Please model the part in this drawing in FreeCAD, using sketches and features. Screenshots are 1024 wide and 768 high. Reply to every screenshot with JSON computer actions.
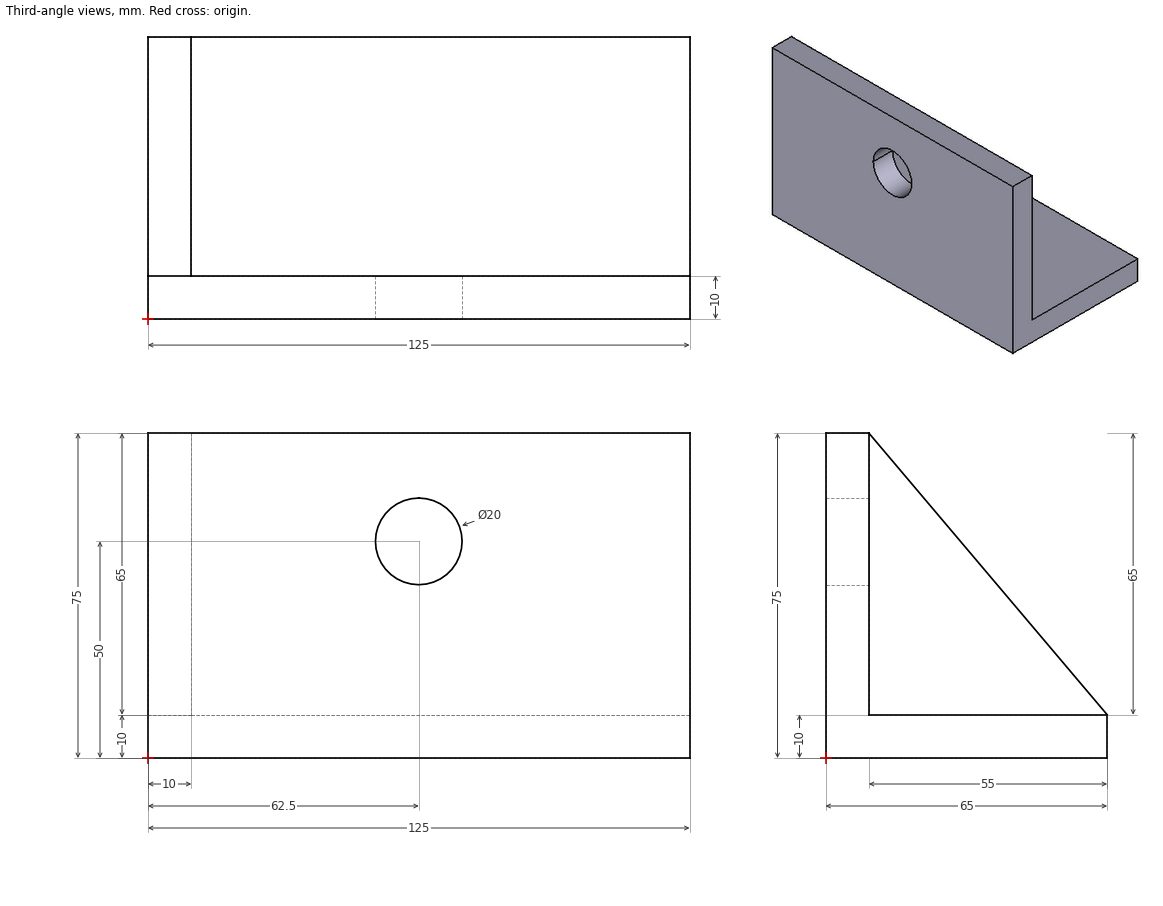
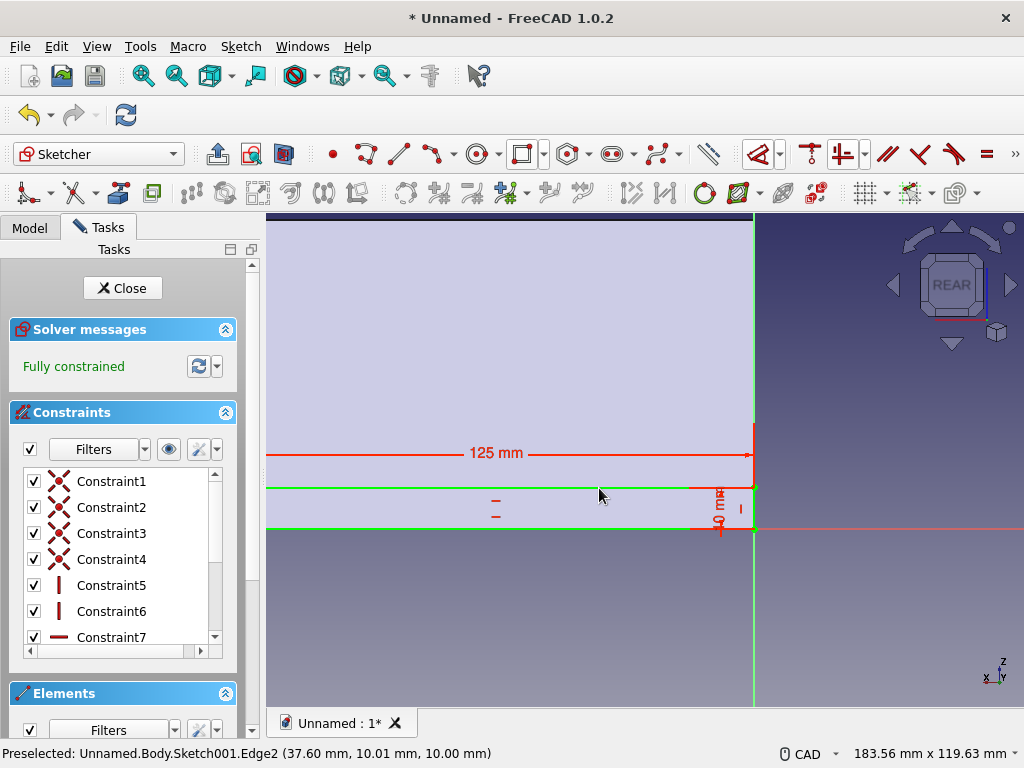
{"action": "left_click", "coordinate": [123, 288]}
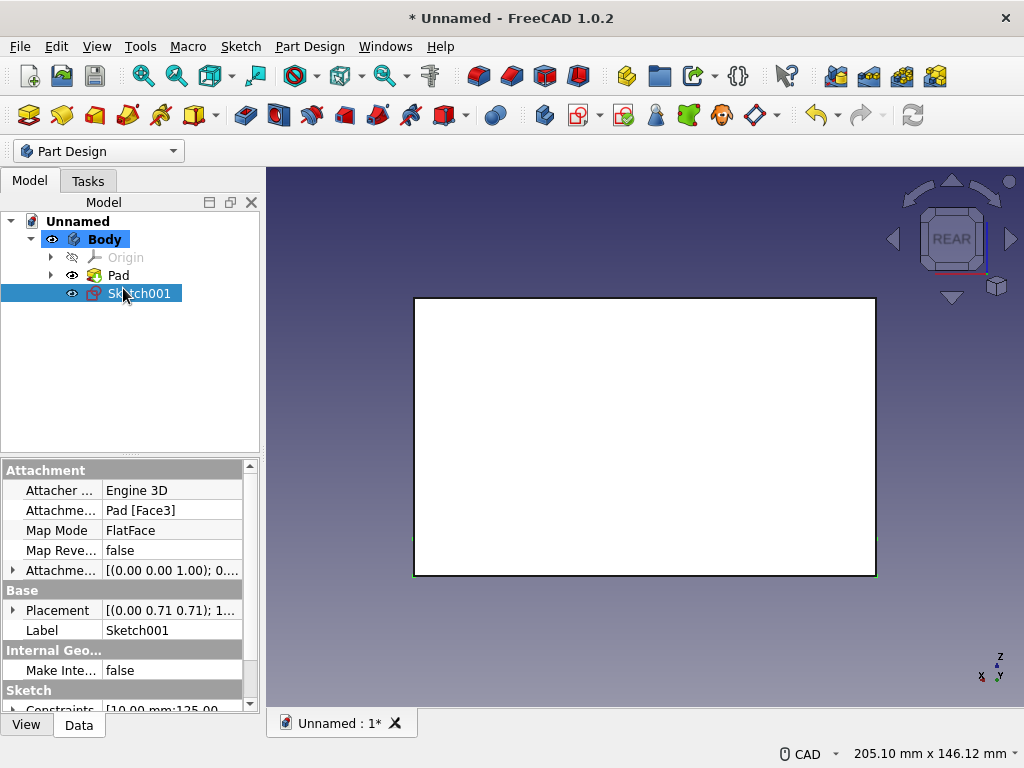
{"action": "left_click", "coordinate": [29, 116]}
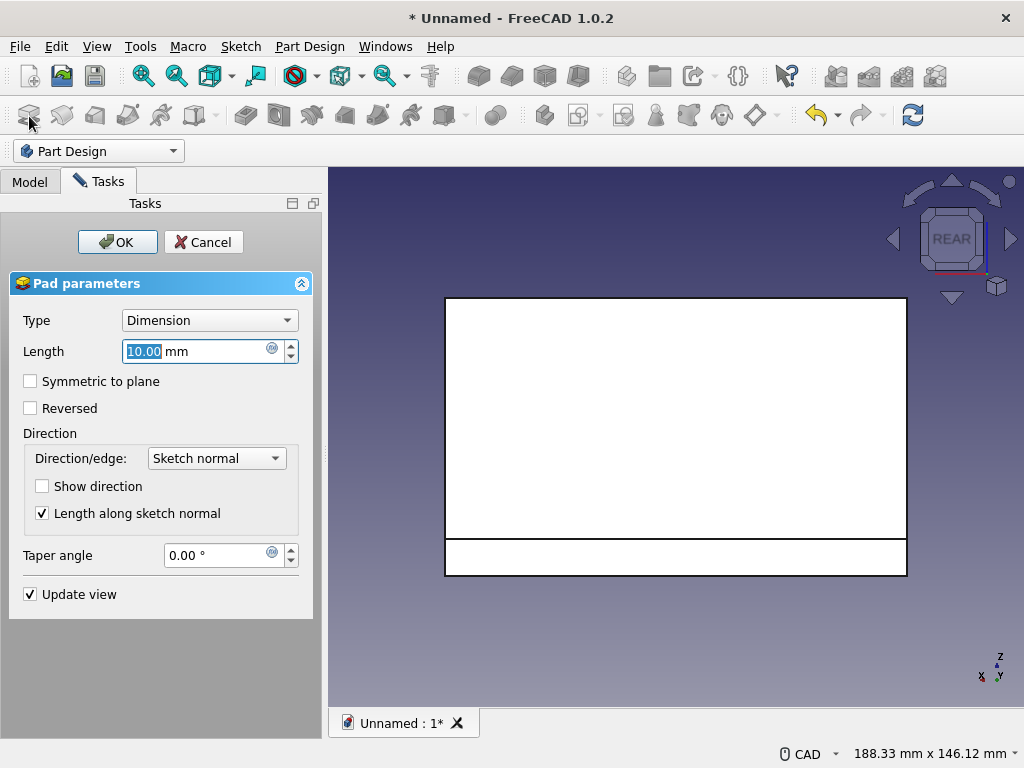
{"action": "type", "text": "55"}
{"action": "key", "text": "Tab"}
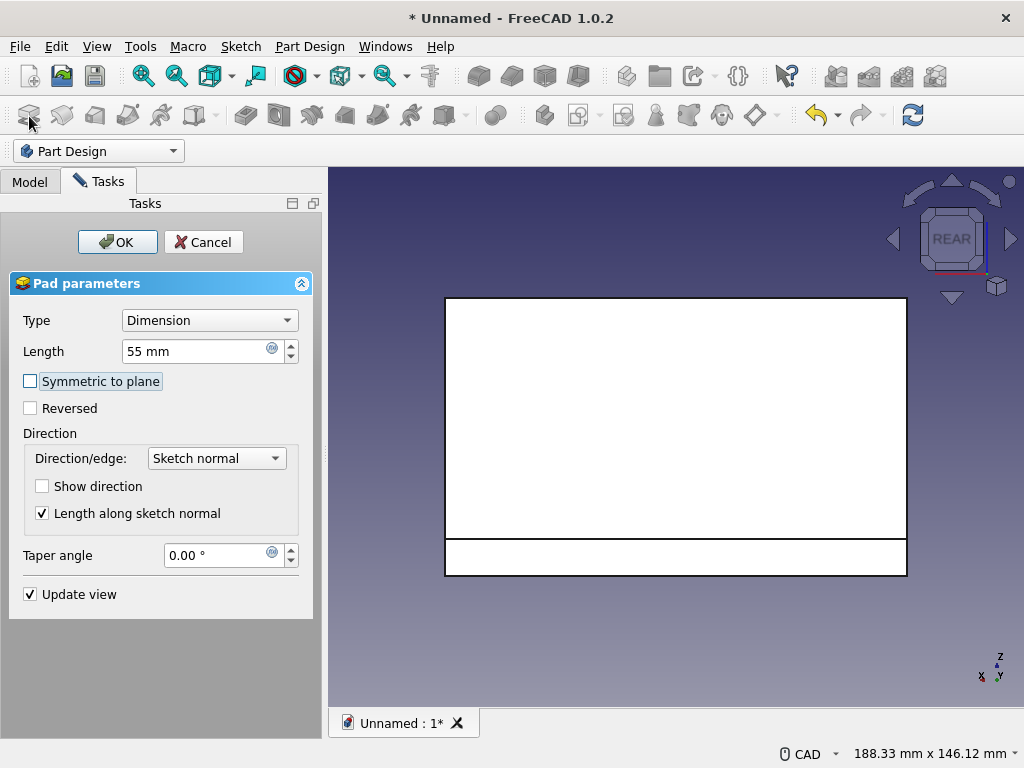
{"action": "left_click", "coordinate": [118, 242]}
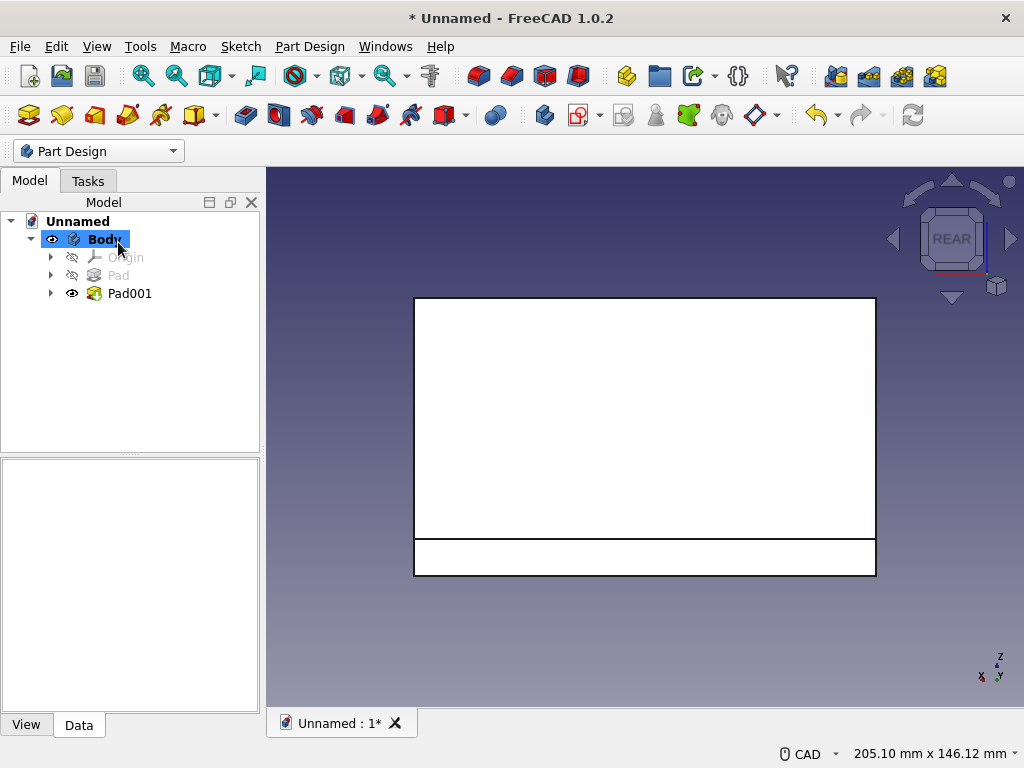
{"action": "left_click", "coordinate": [579, 418]}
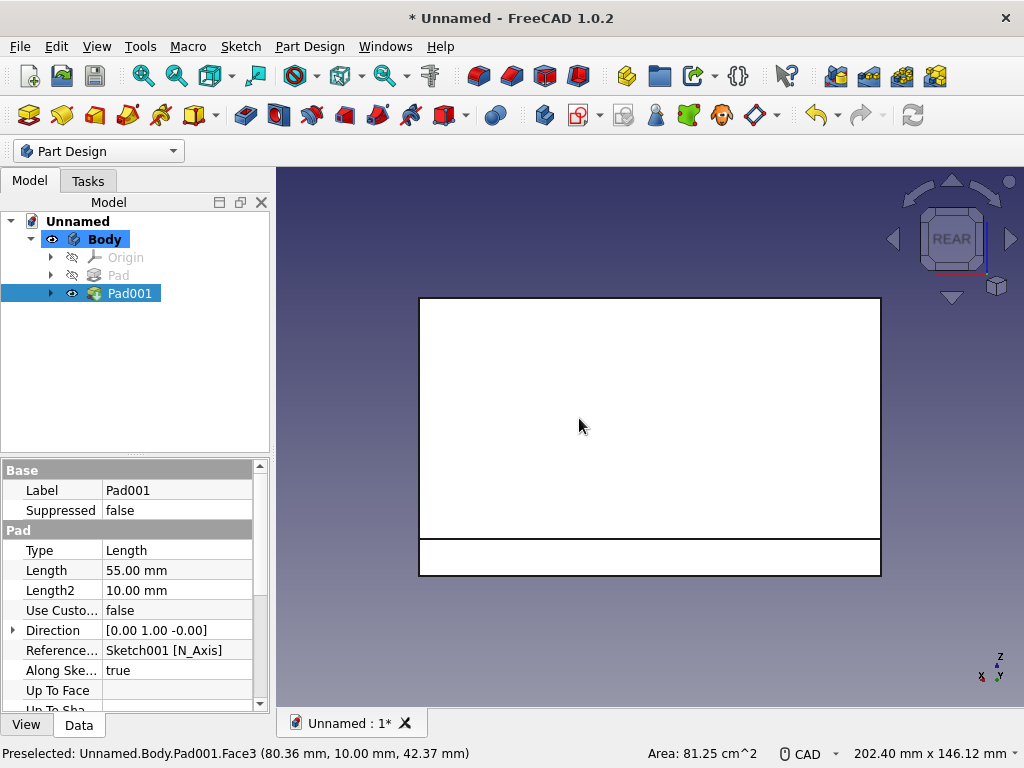
{"action": "left_click", "coordinate": [578, 116]}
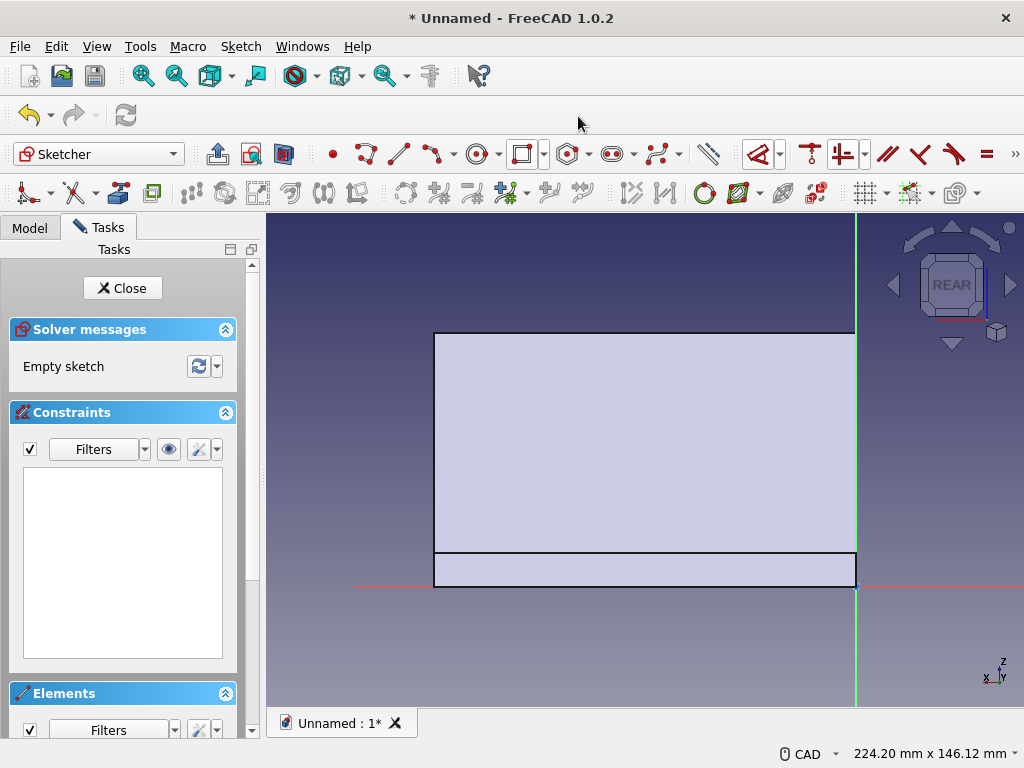
{"action": "key", "text": "q s"}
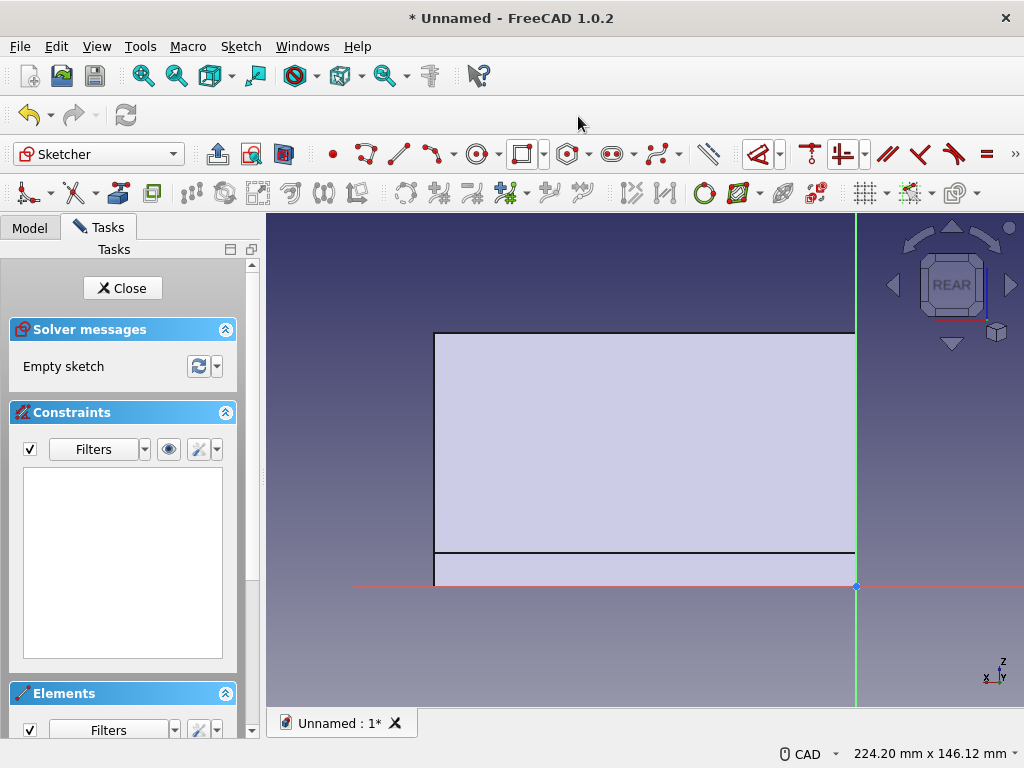
{"action": "scroll", "coordinate": [294, 460], "scroll_direction": "down", "scroll_amount": 1}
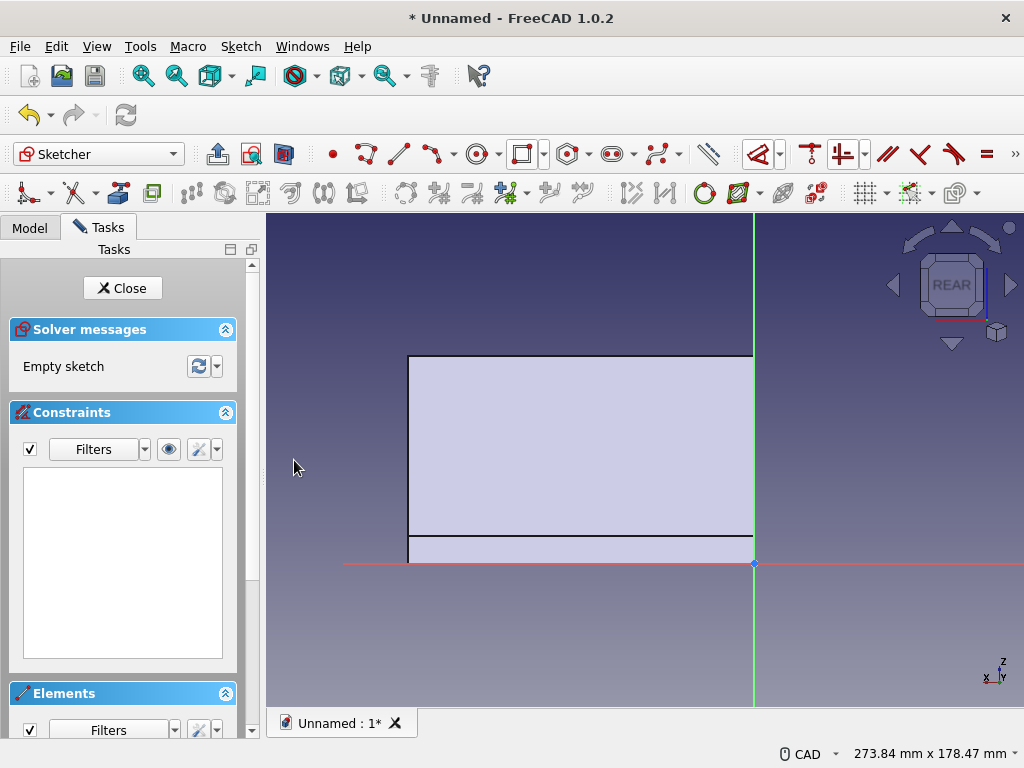
{"action": "scroll", "coordinate": [859, 460], "scroll_direction": "up", "scroll_amount": 2}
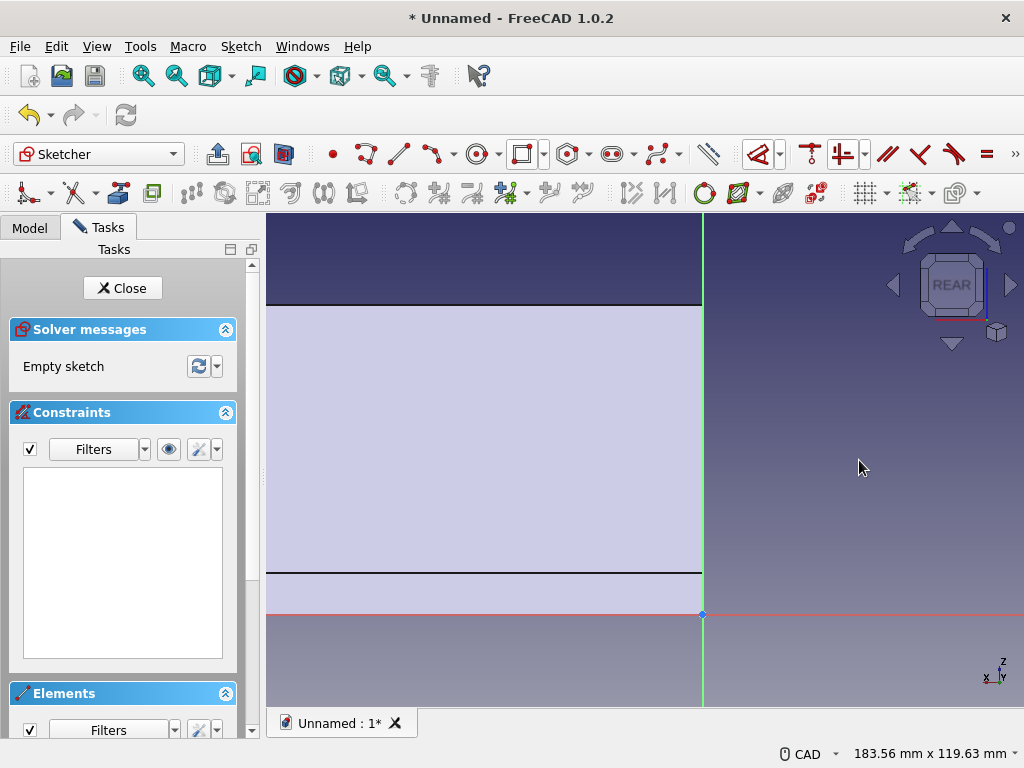
{"action": "left_click", "coordinate": [522, 154]}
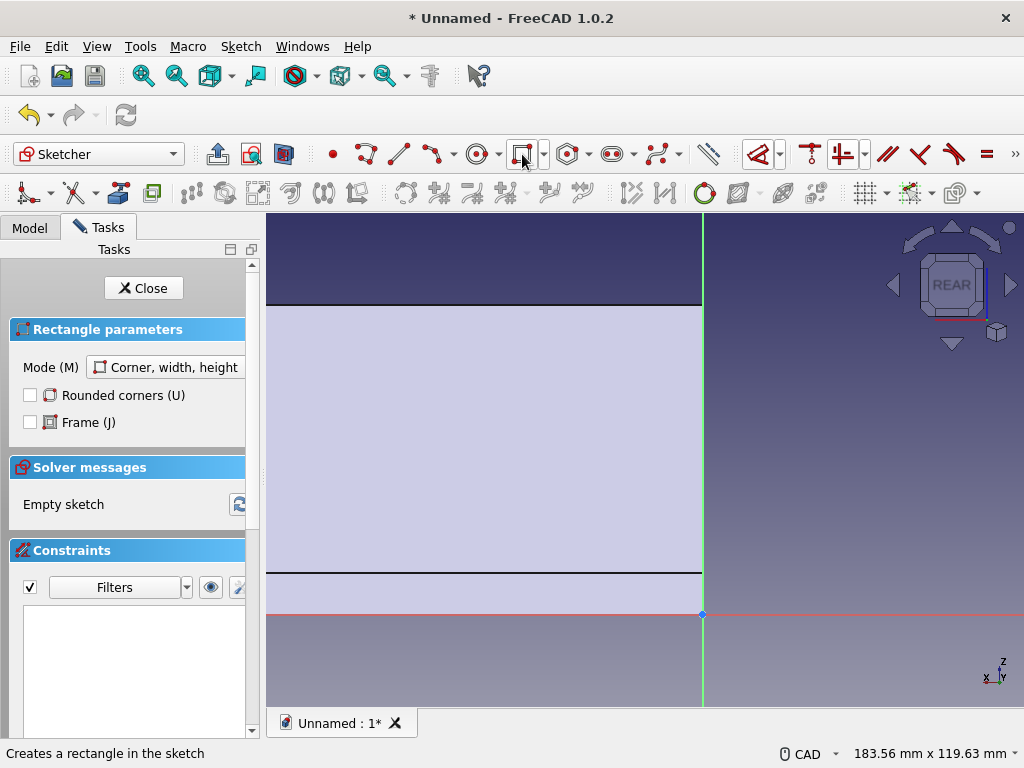
{"action": "left_click", "coordinate": [661, 305]}
{"action": "left_click", "coordinate": [703, 573]}
{"action": "key", "text": "Escape"}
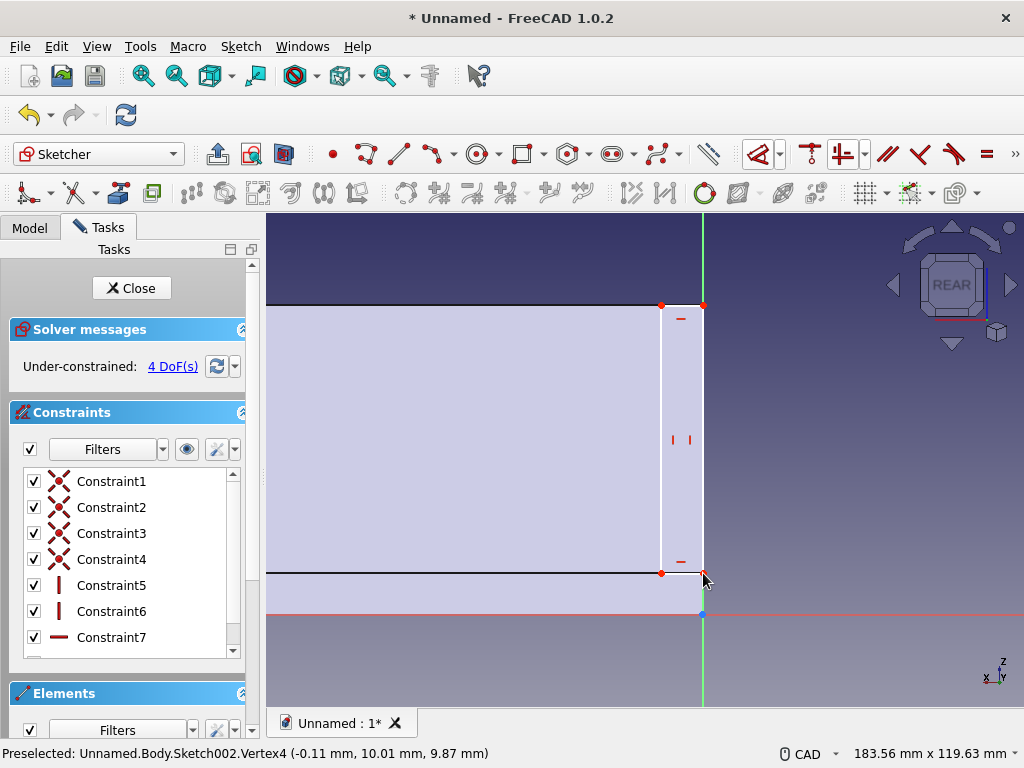
{"action": "left_click", "coordinate": [703, 574]}